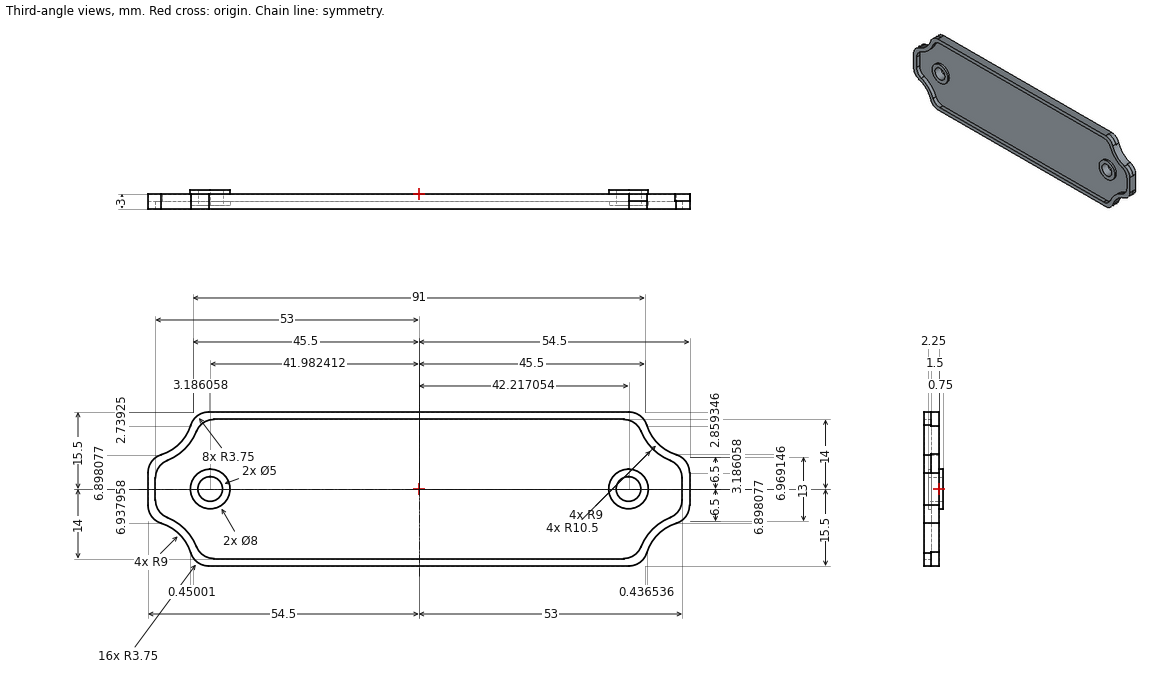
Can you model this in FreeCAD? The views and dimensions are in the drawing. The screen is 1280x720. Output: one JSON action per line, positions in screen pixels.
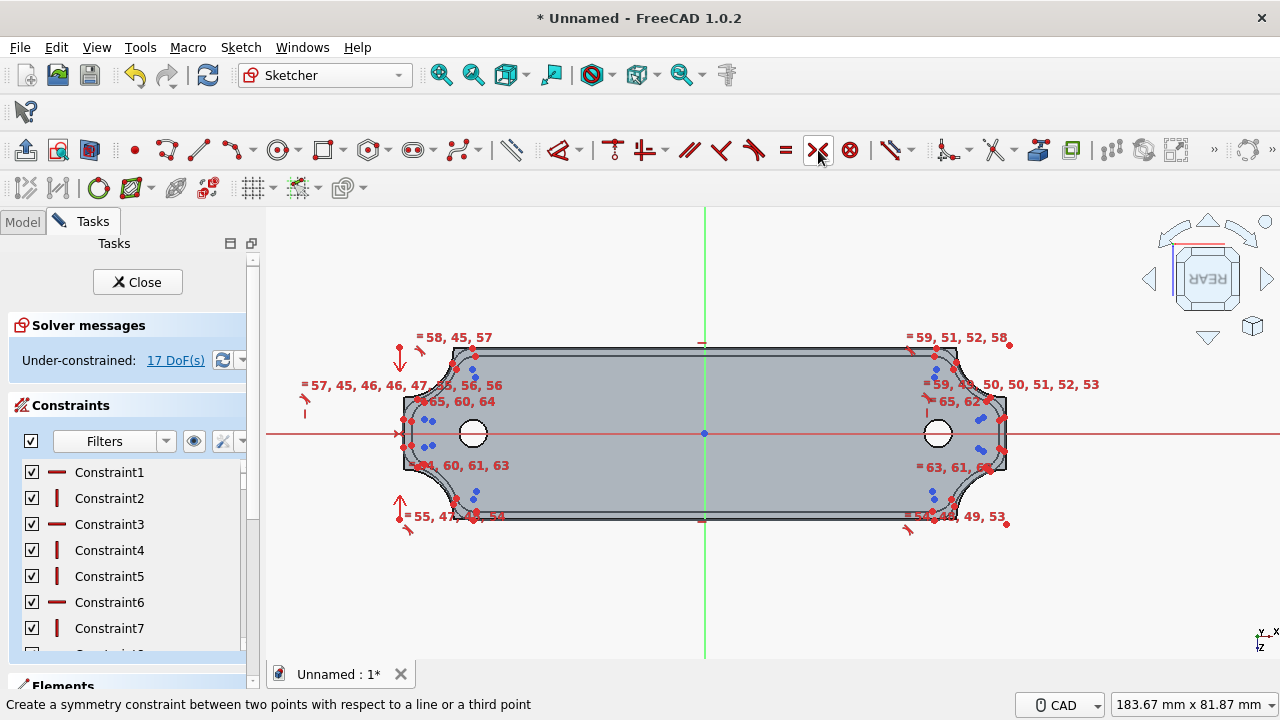
{"action": "left_click", "coordinate": [400, 520]}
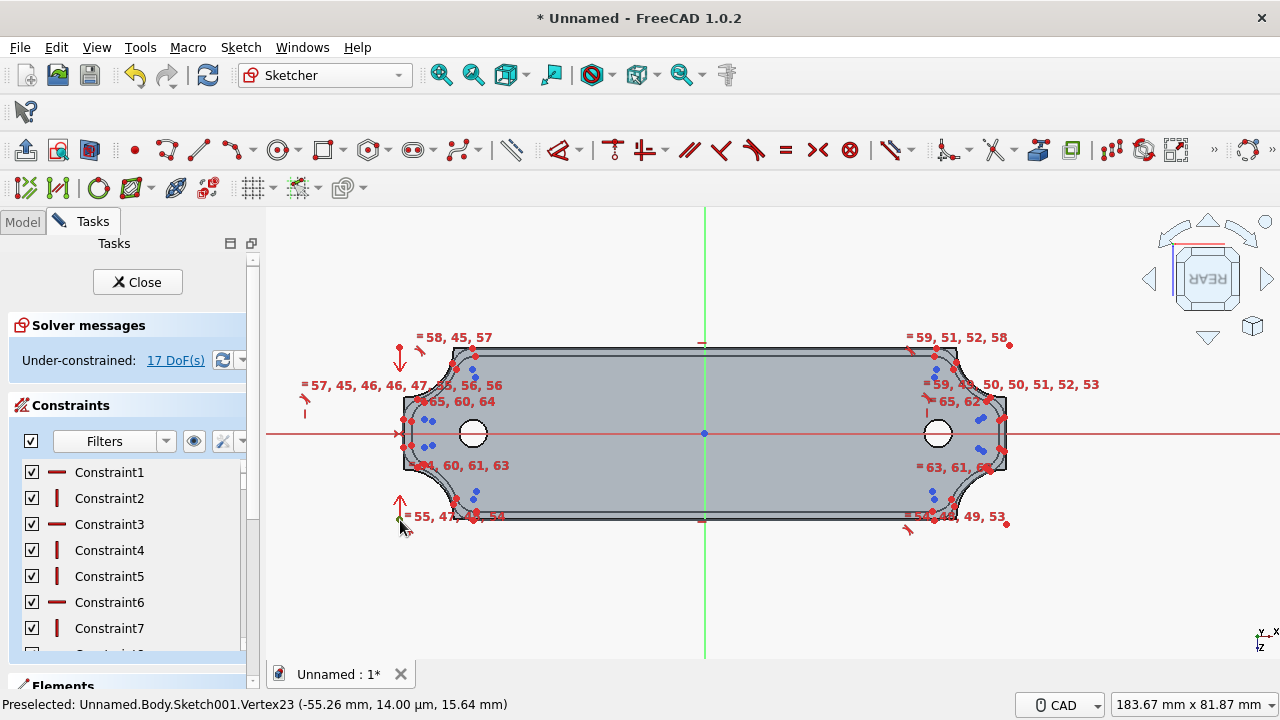
{"action": "left_click", "coordinate": [1007, 525]}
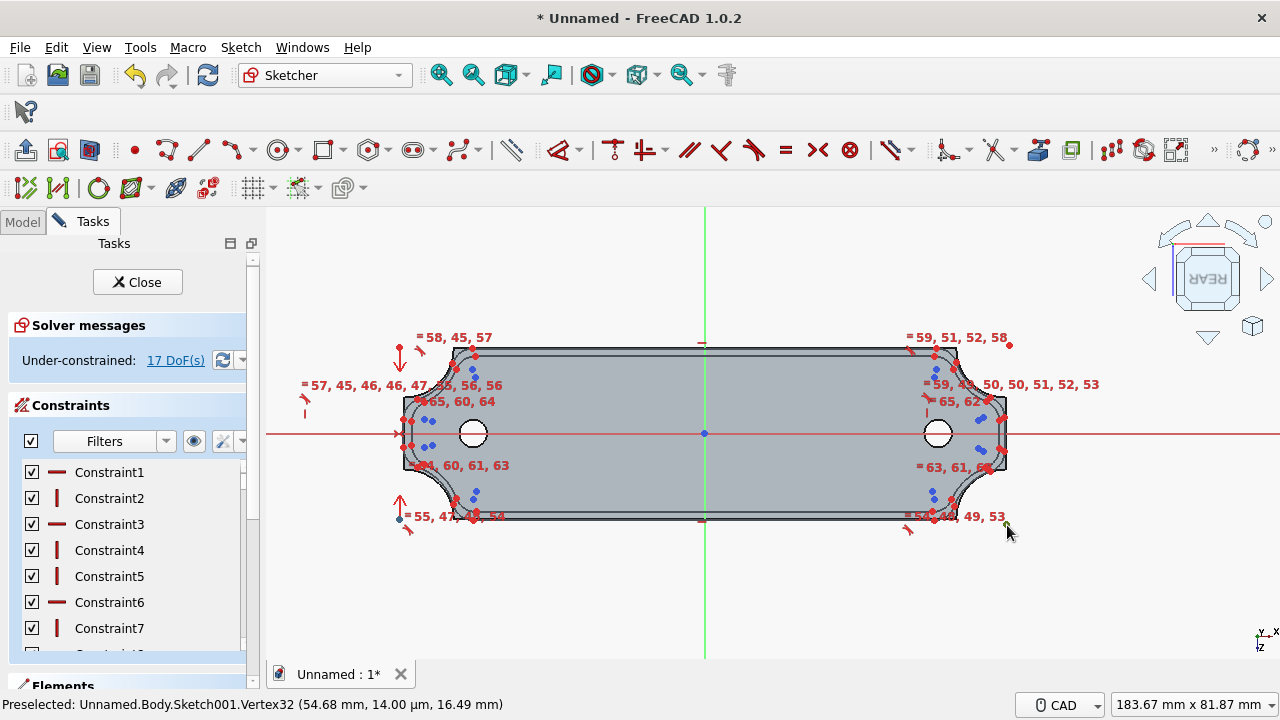
{"action": "left_click", "coordinate": [705, 603]}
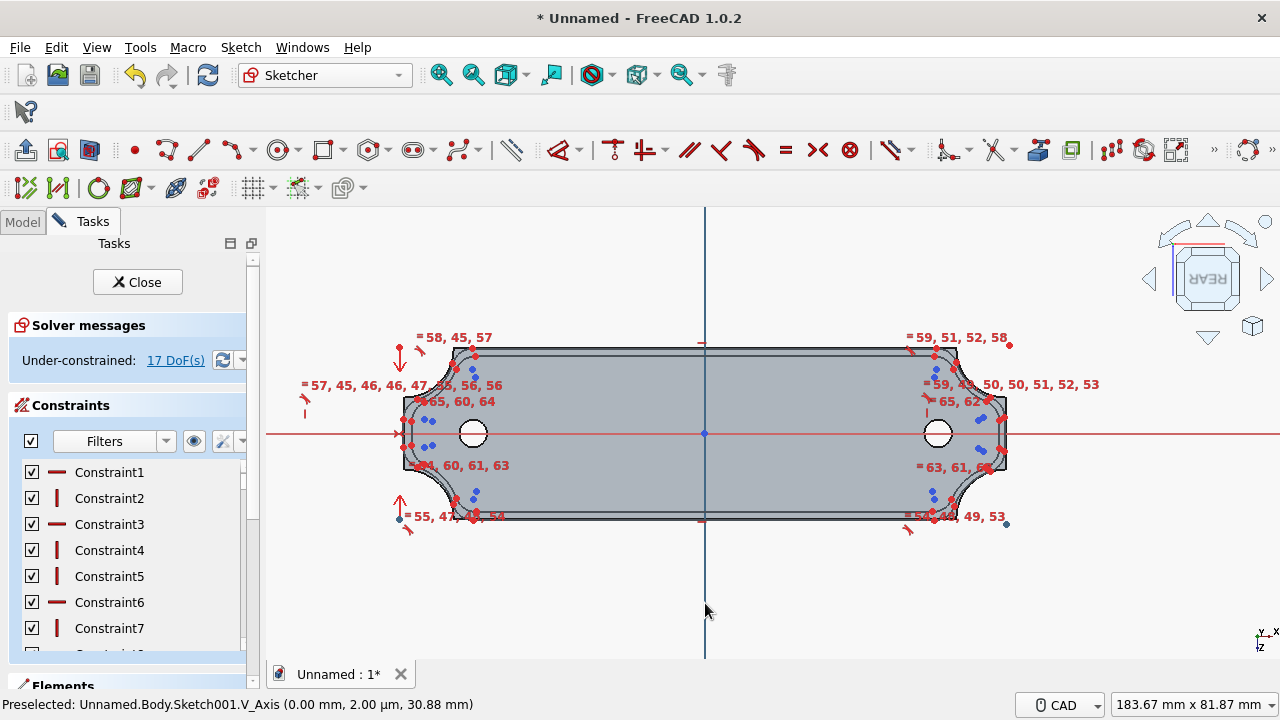
{"action": "left_click", "coordinate": [818, 150]}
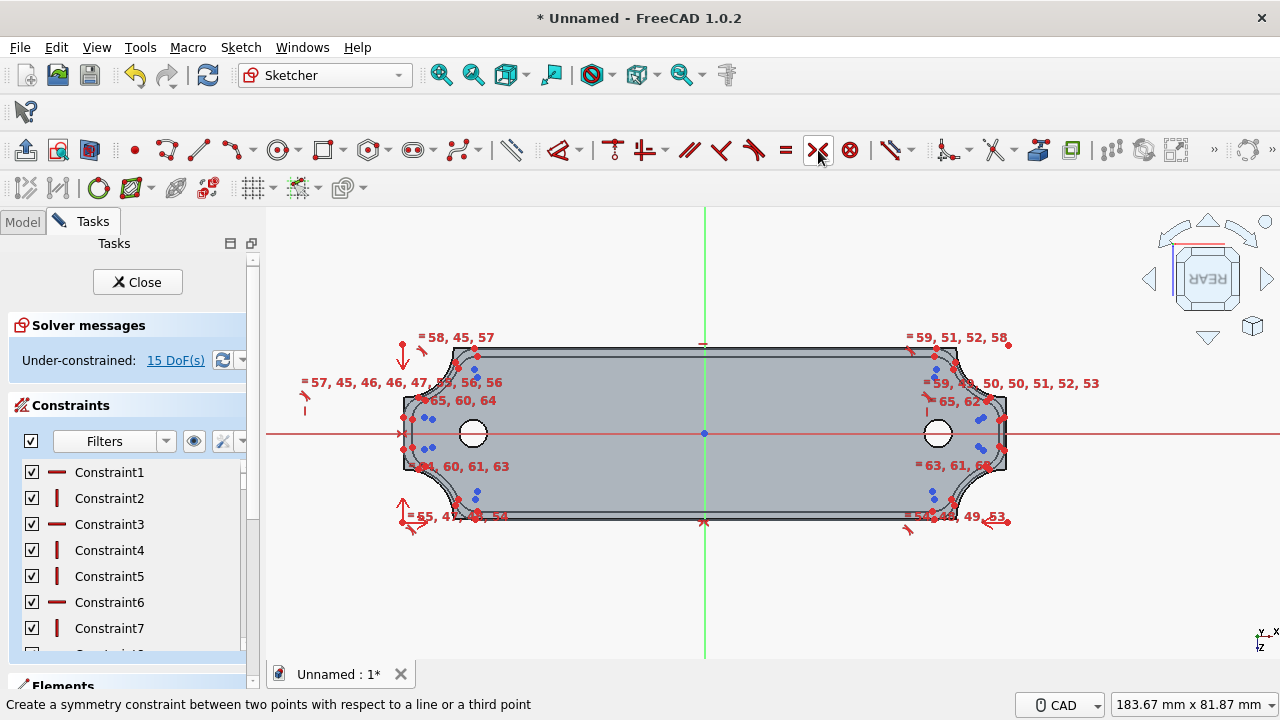
{"action": "scroll", "coordinate": [424, 418], "scroll_direction": "up", "scroll_amount": 2}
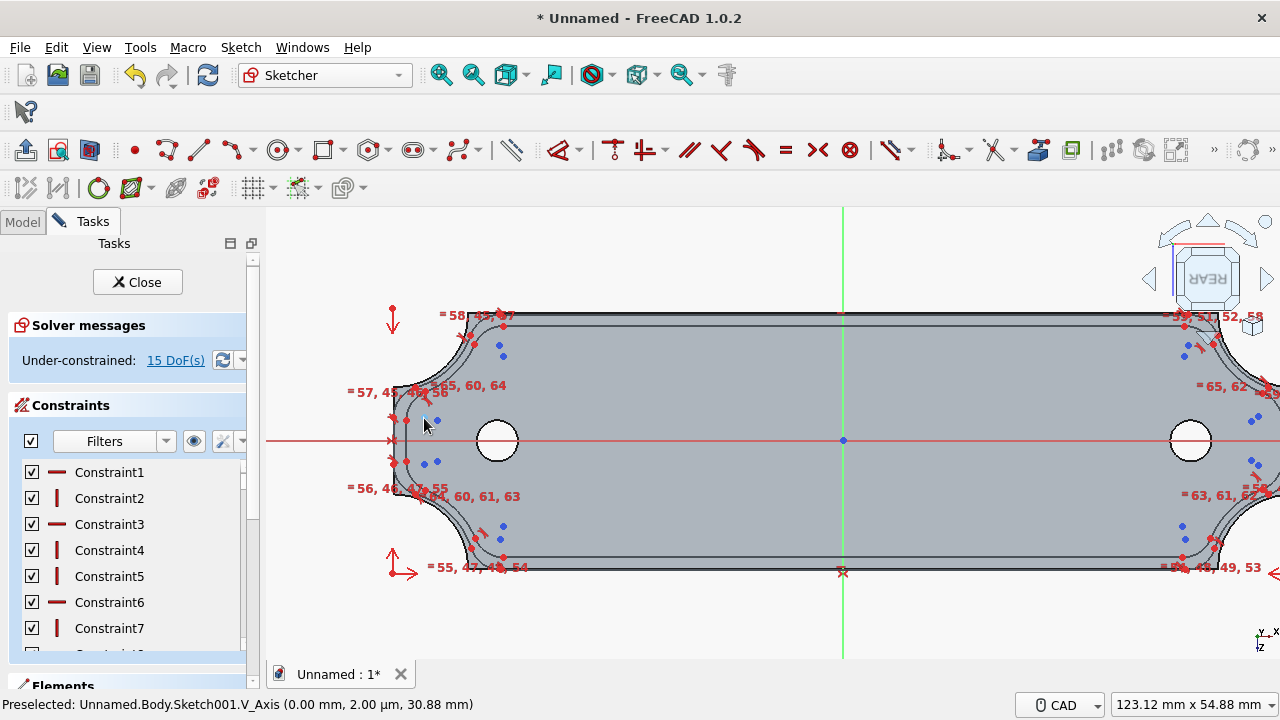
{"action": "left_click", "coordinate": [424, 417]}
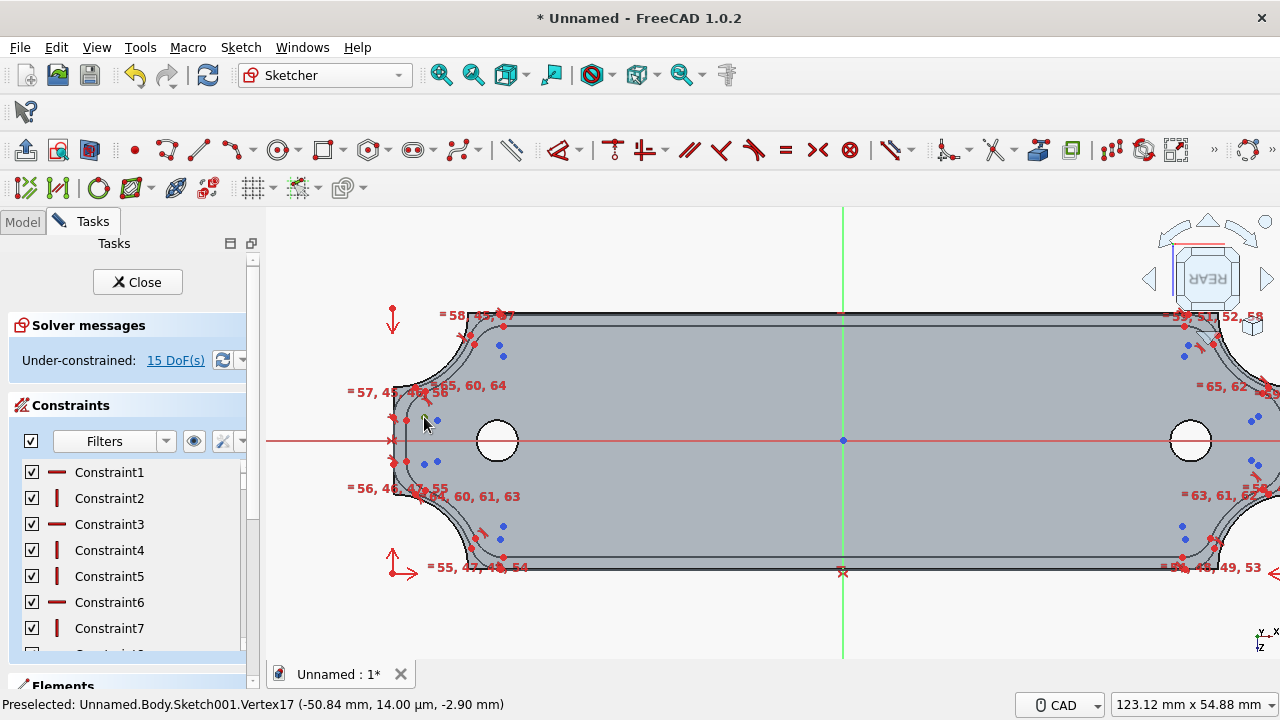
{"action": "scroll", "coordinate": [423, 417], "scroll_direction": "down", "scroll_amount": 2}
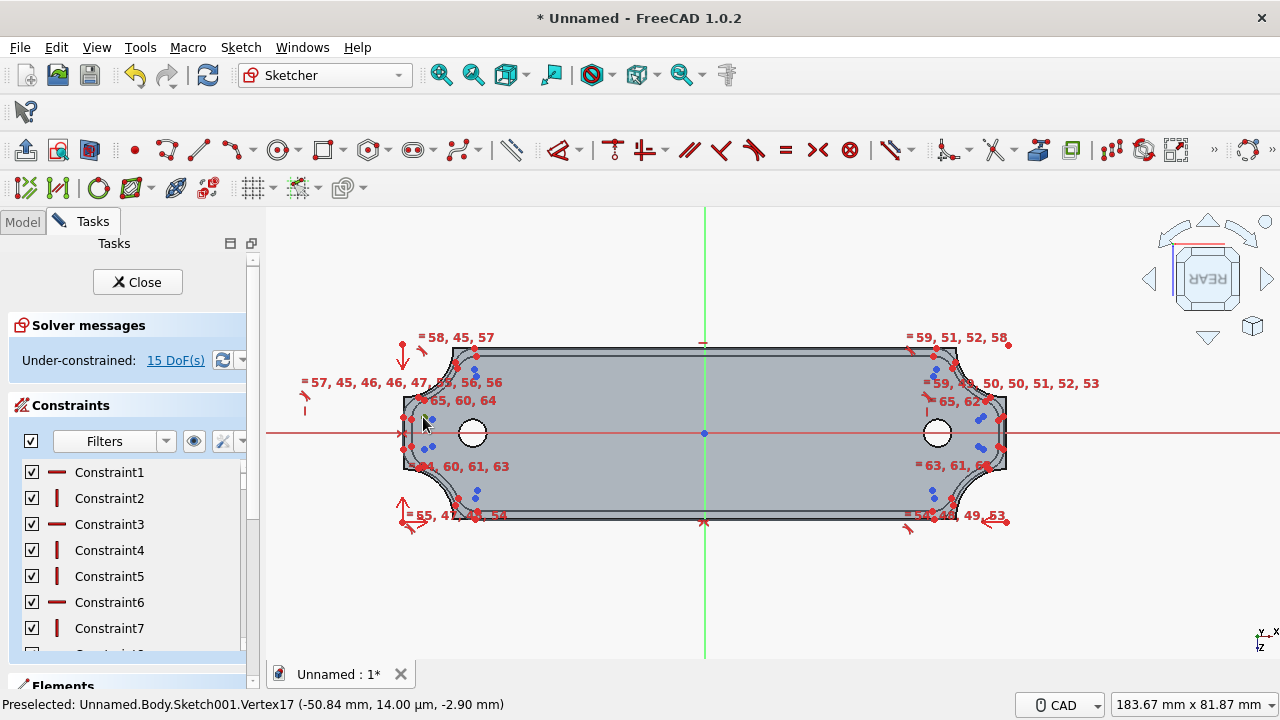
{"action": "scroll", "coordinate": [983, 417], "scroll_direction": "up", "scroll_amount": 4}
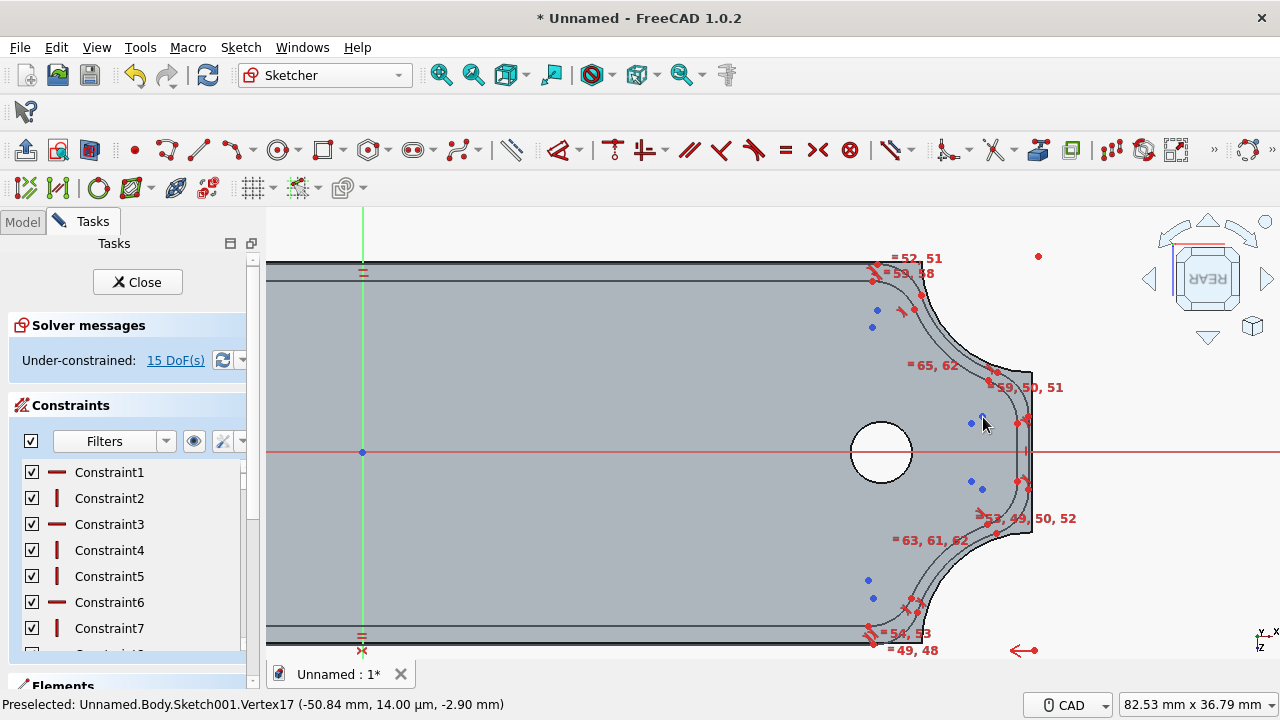
{"action": "left_click", "coordinate": [983, 416]}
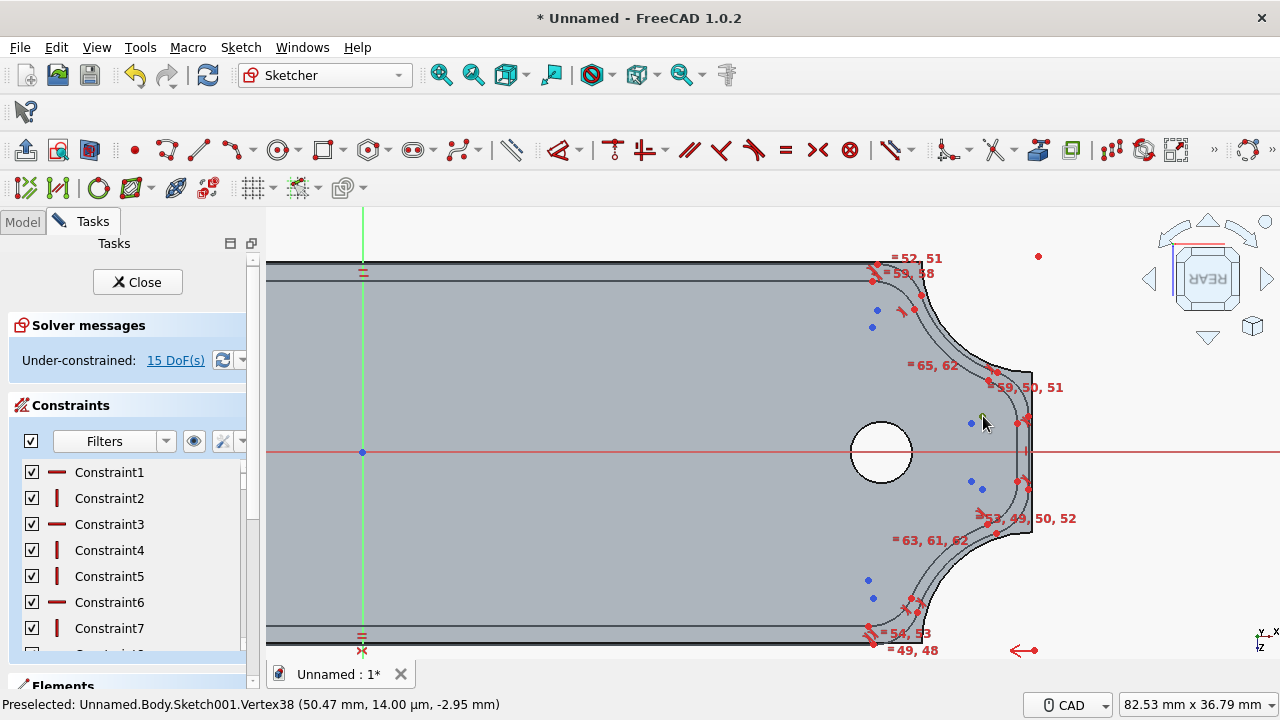
{"action": "left_click", "coordinate": [363, 574]}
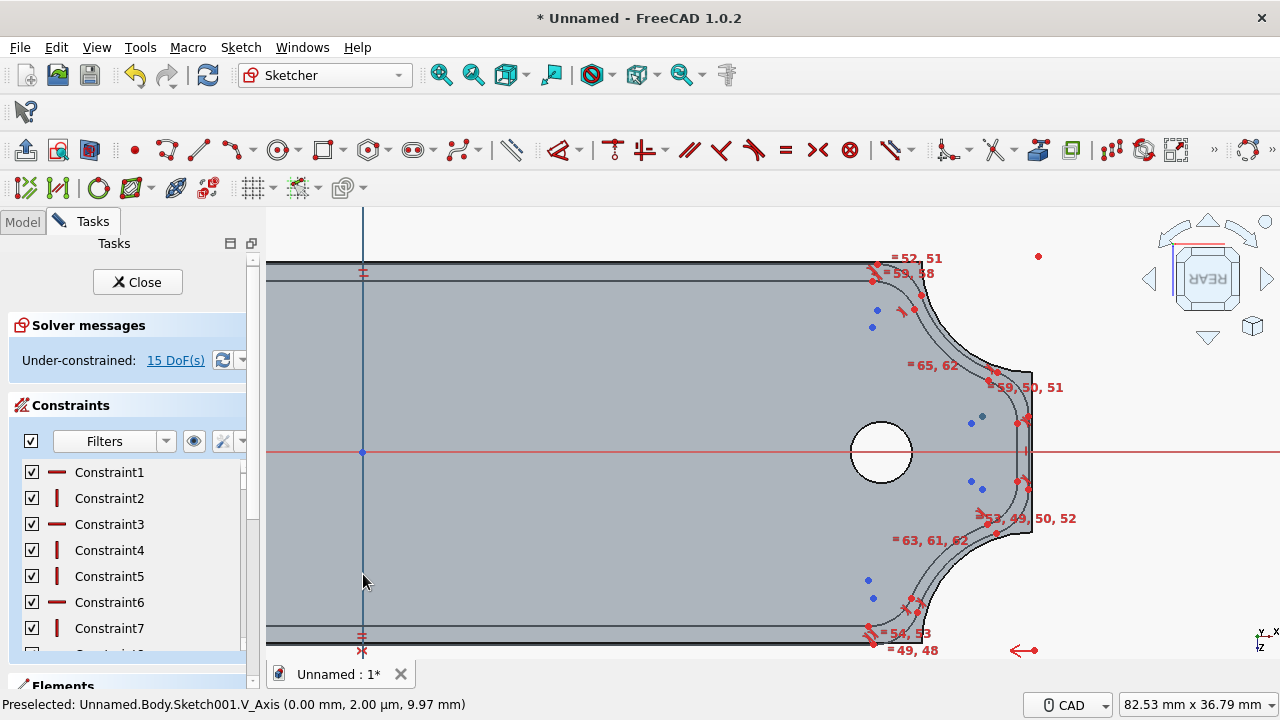
{"action": "left_click", "coordinate": [818, 150]}